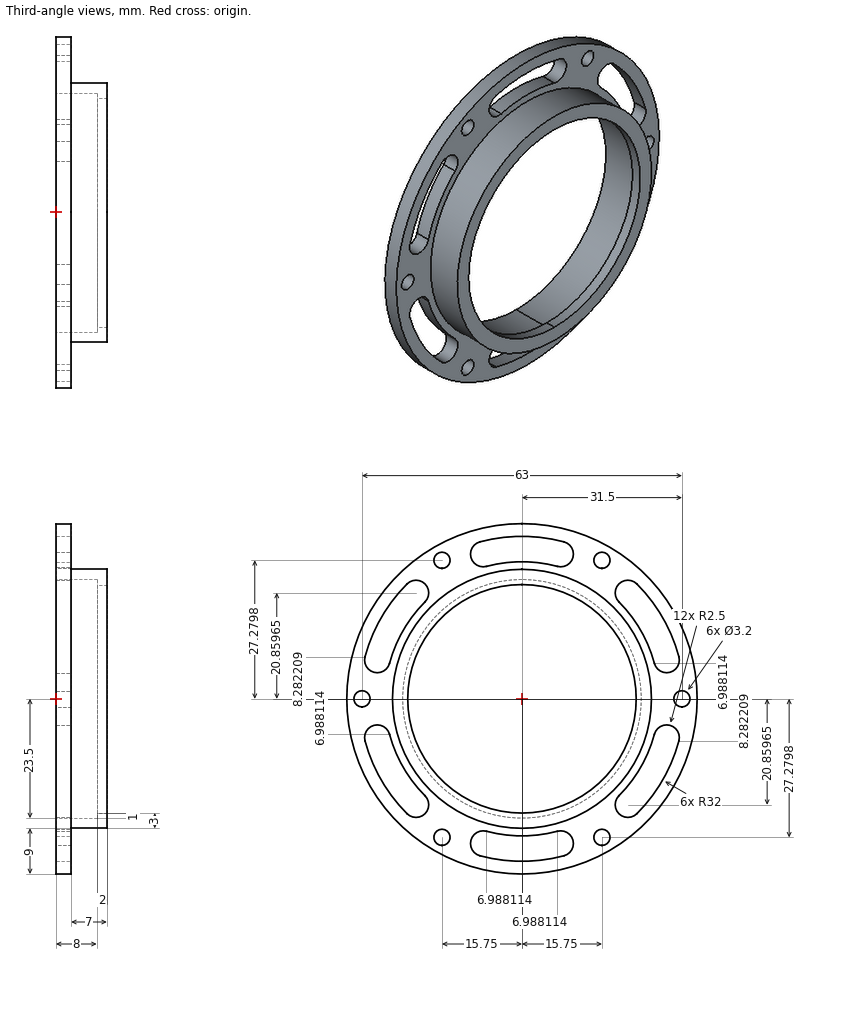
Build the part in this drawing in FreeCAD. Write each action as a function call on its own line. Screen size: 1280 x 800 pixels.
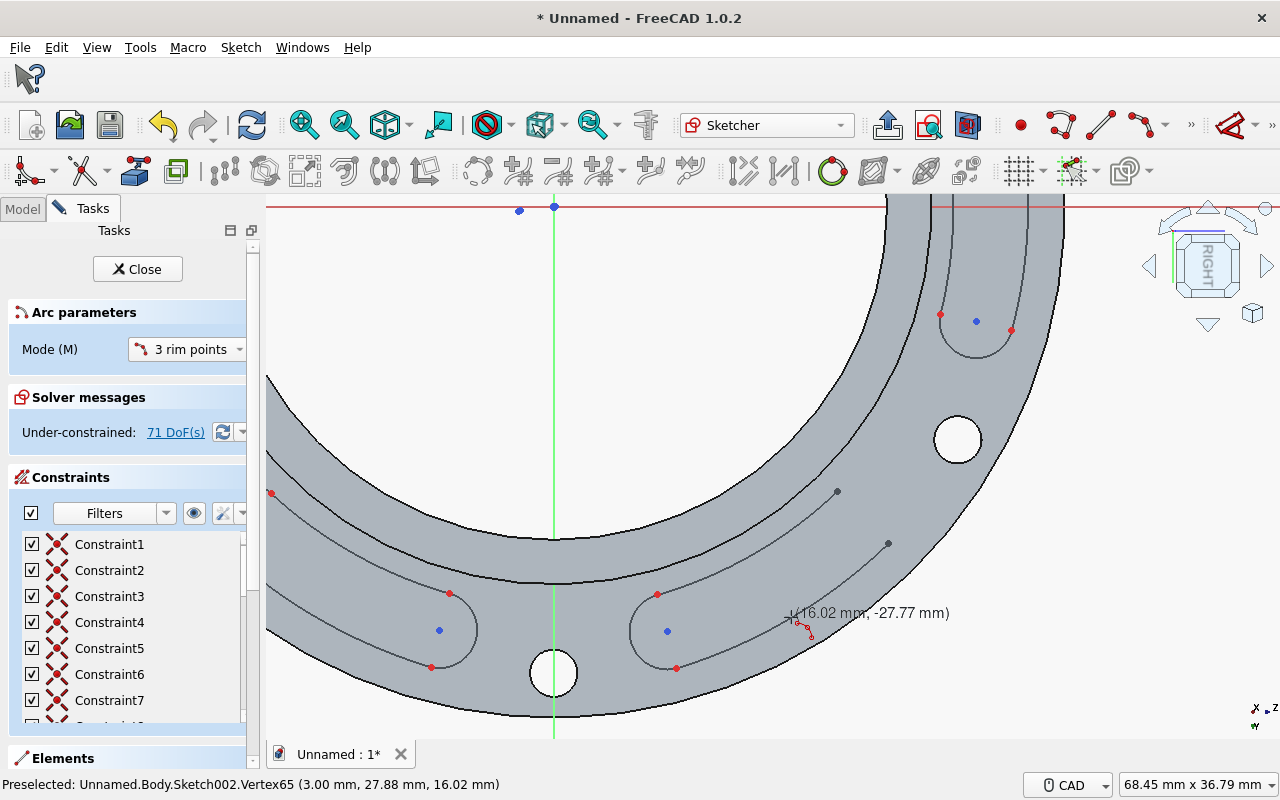
click(889, 543)
click(837, 492)
click(889, 489)
key(Escape)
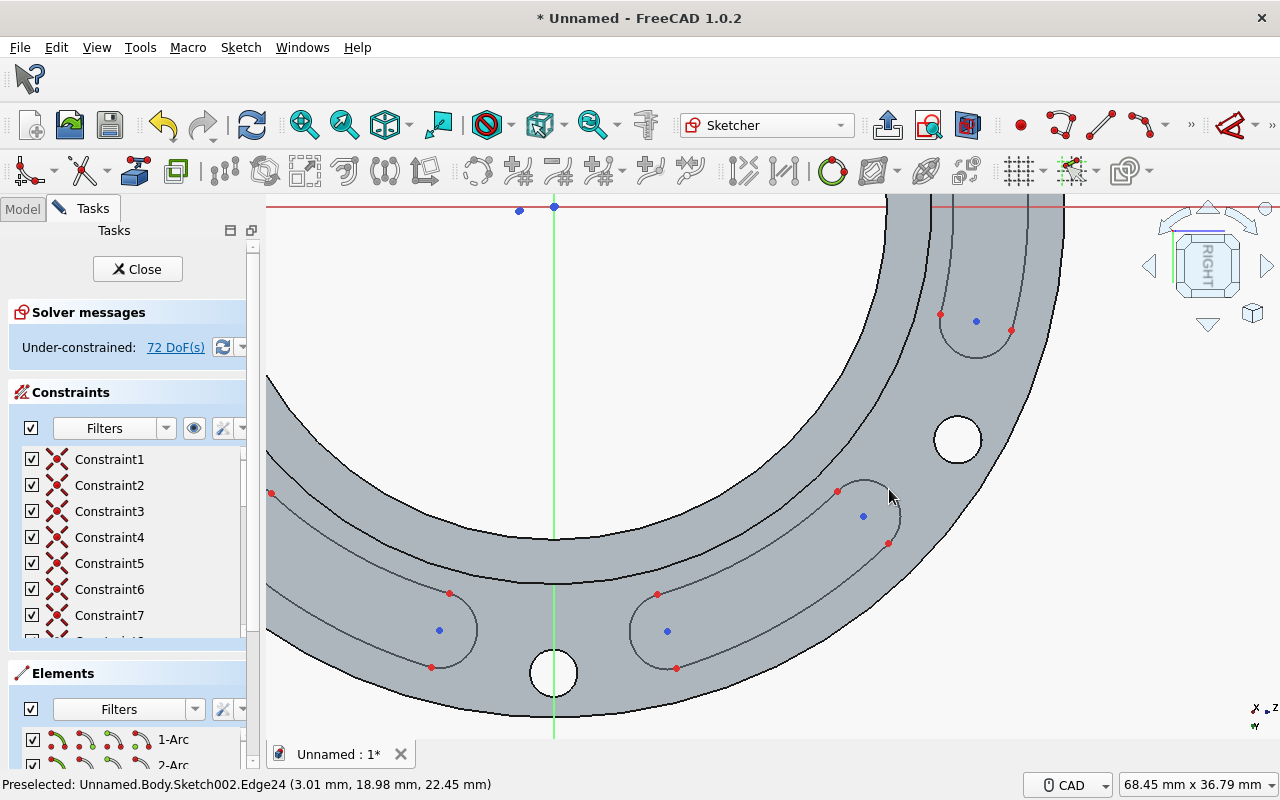
scroll(792, 618, down, 5)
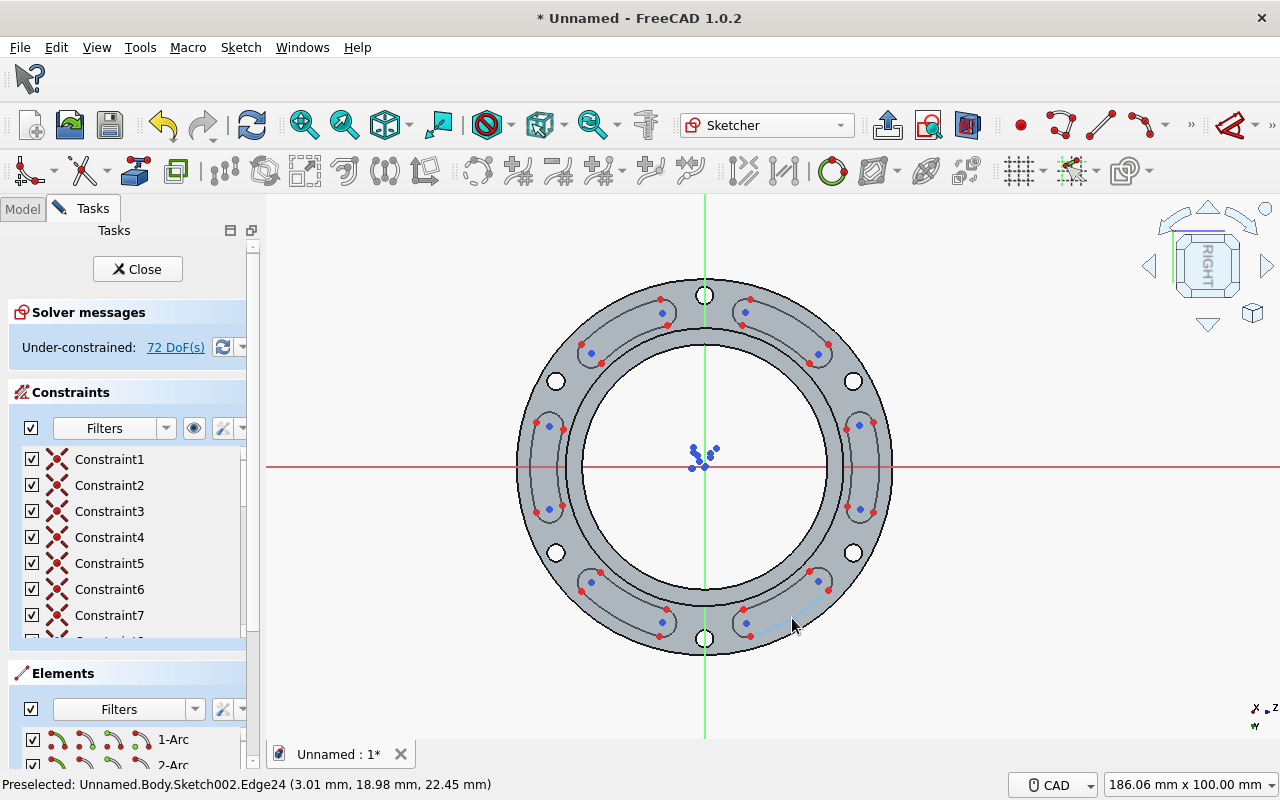
click(589, 569)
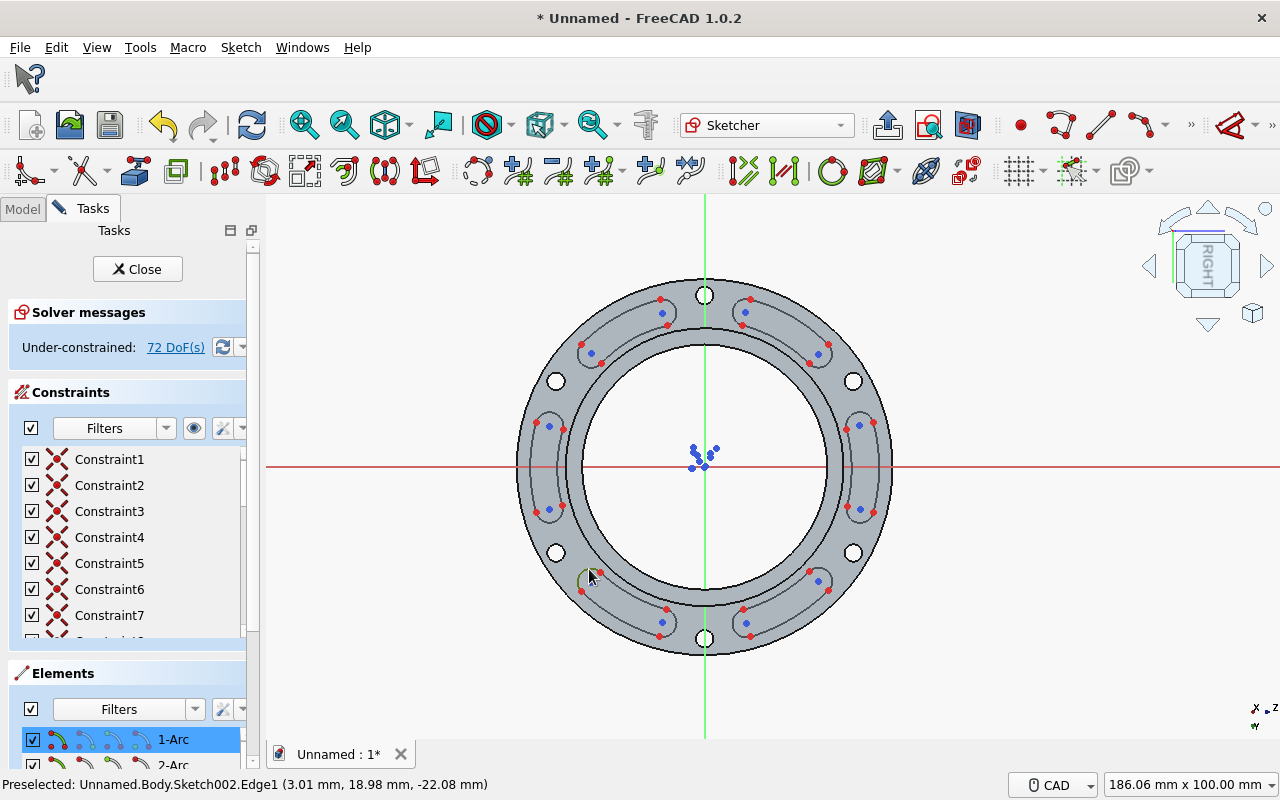
click(603, 609)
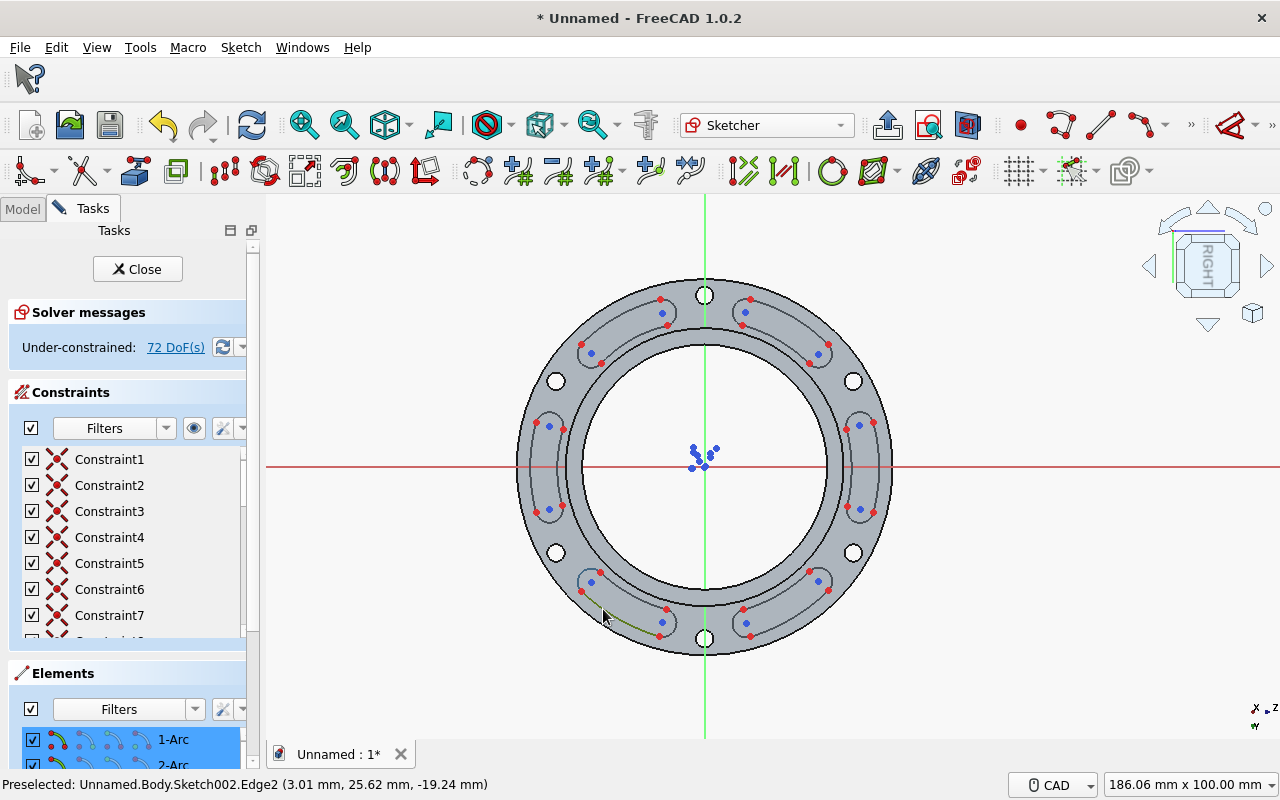
key(t)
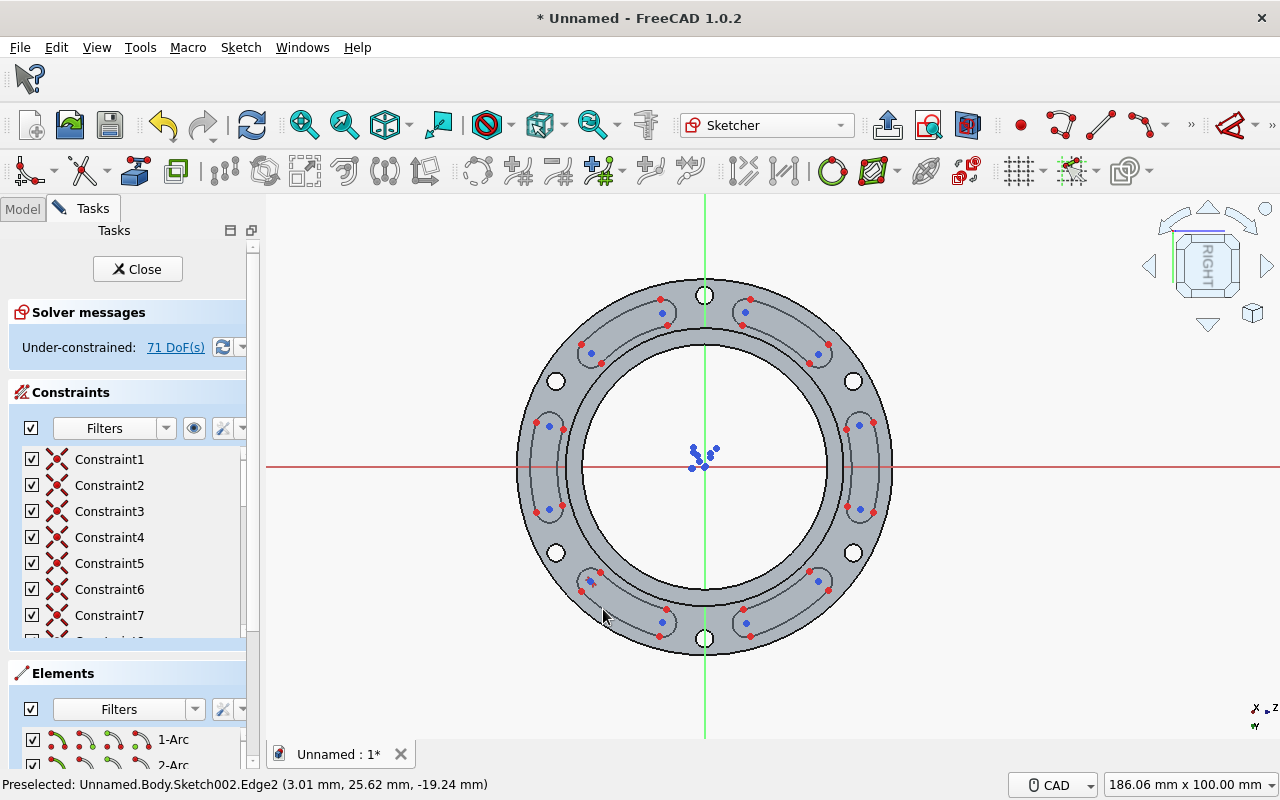
click(589, 569)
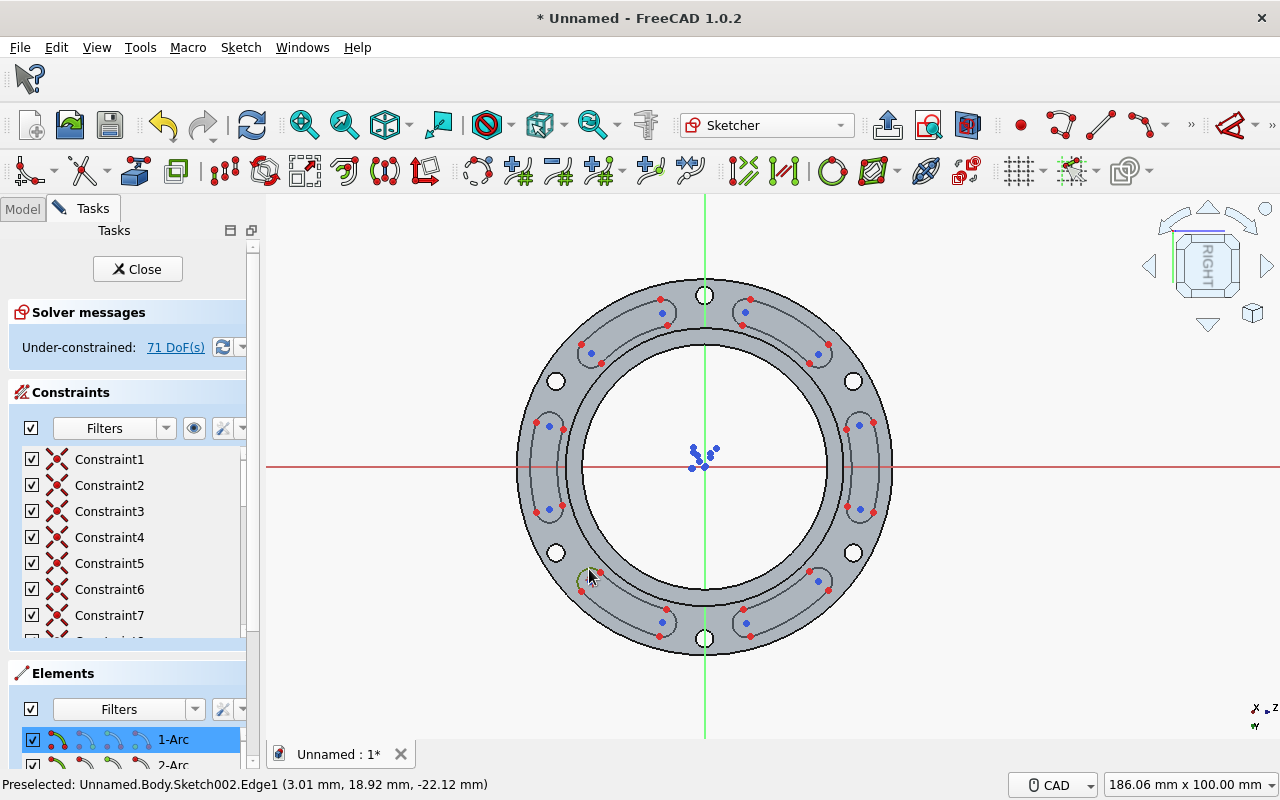
click(618, 587)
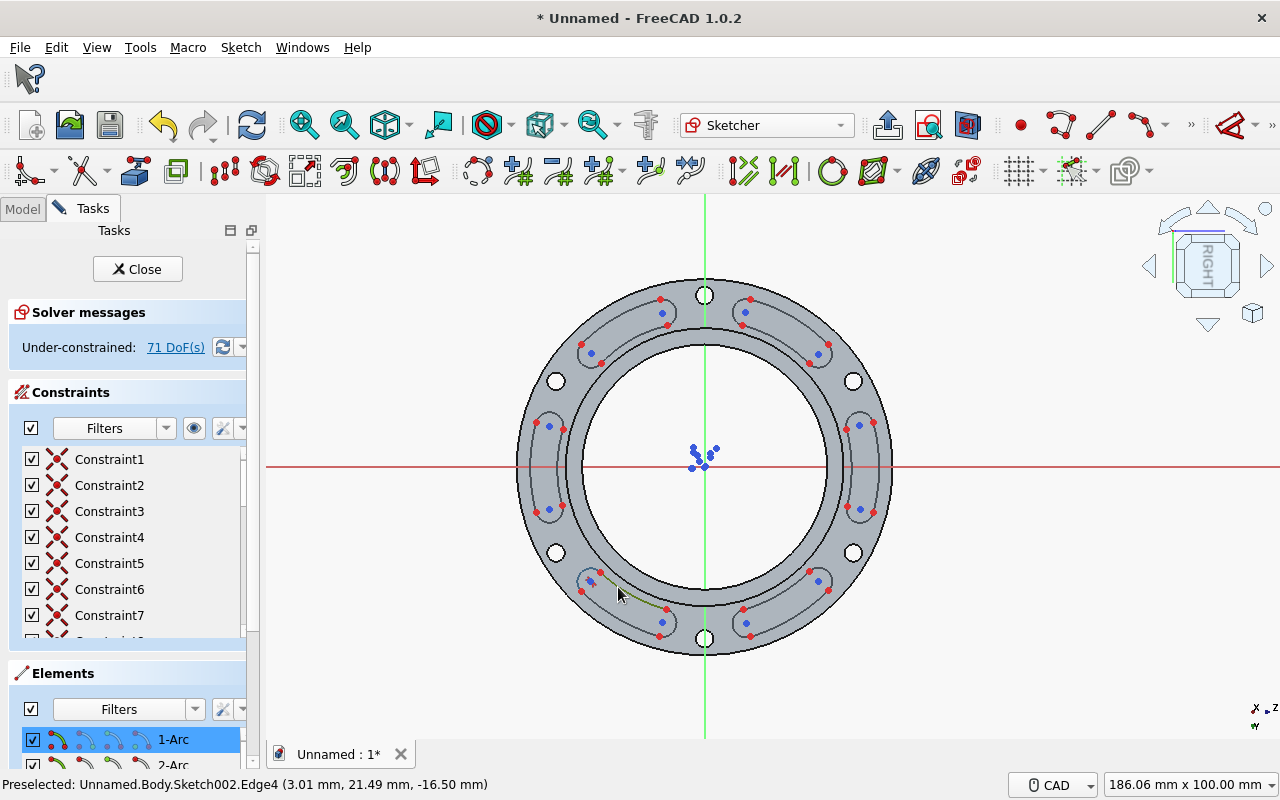
key(t)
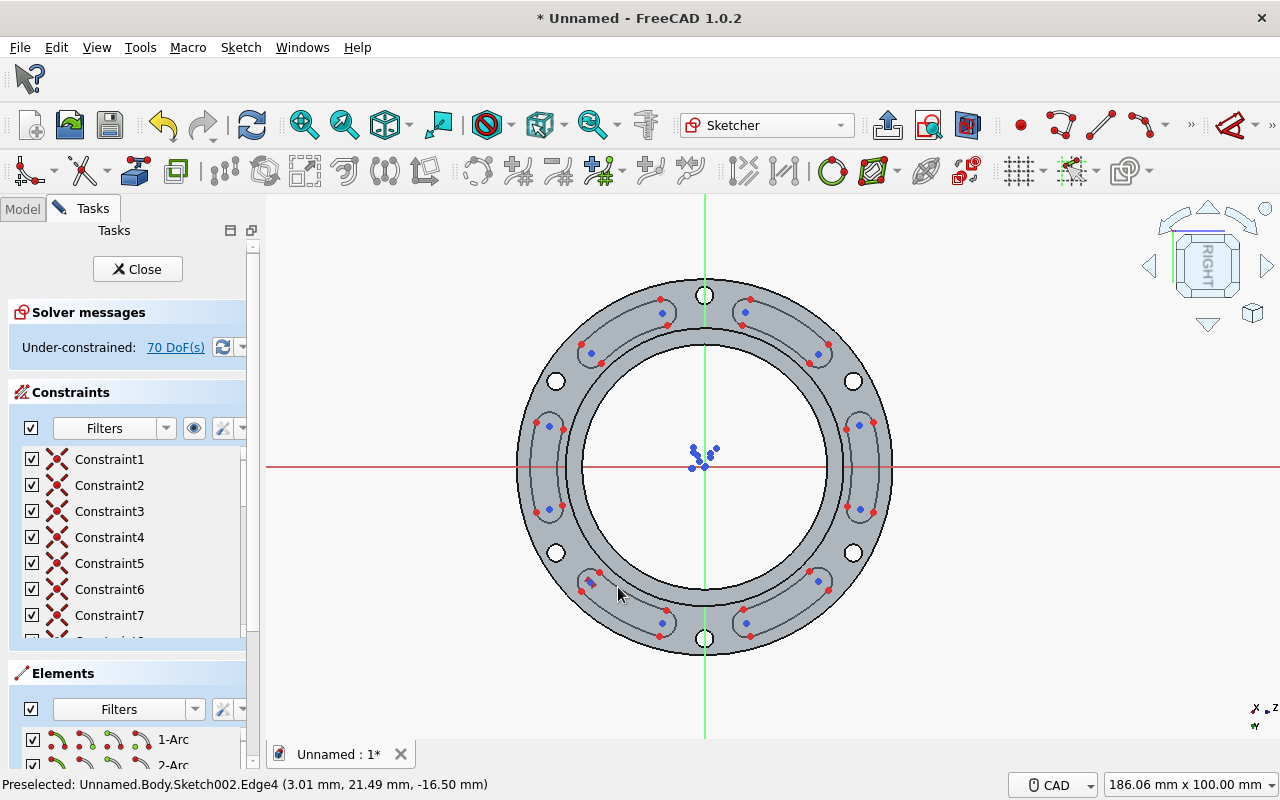
click(603, 609)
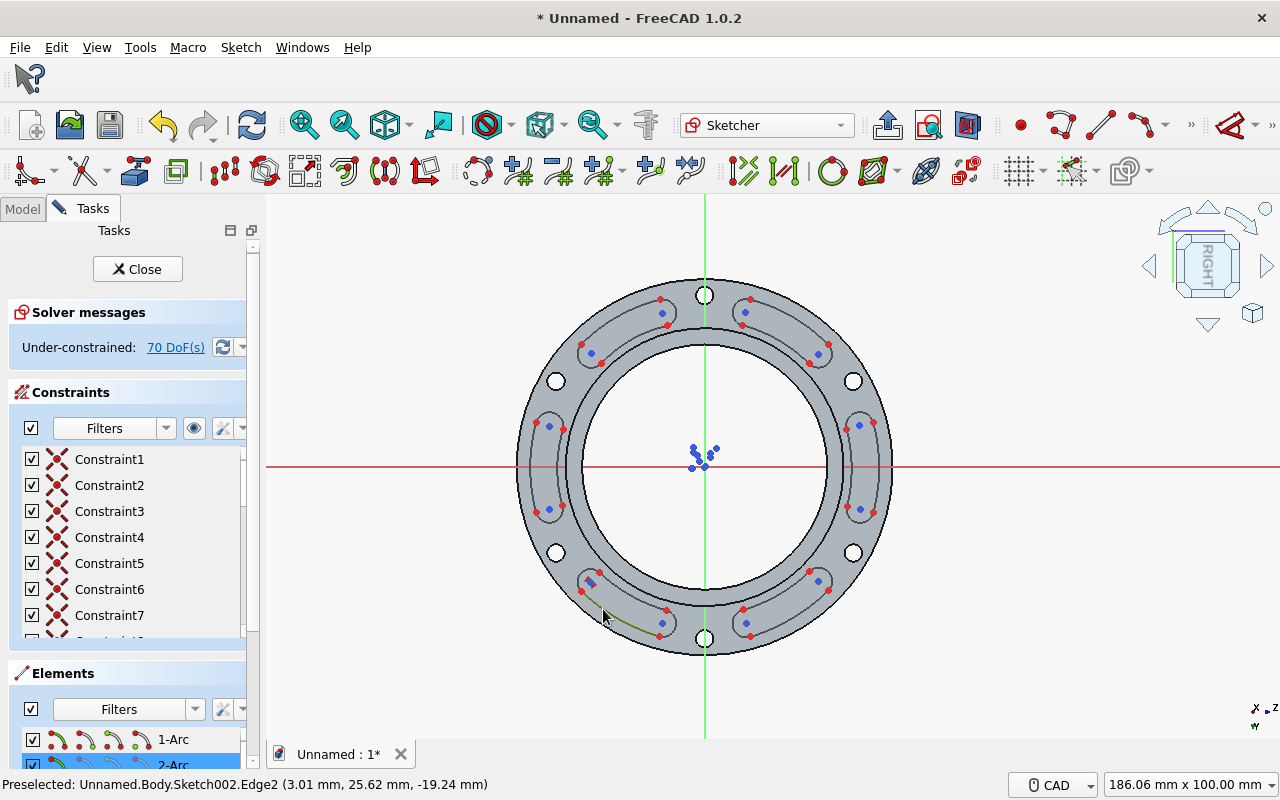
click(671, 634)